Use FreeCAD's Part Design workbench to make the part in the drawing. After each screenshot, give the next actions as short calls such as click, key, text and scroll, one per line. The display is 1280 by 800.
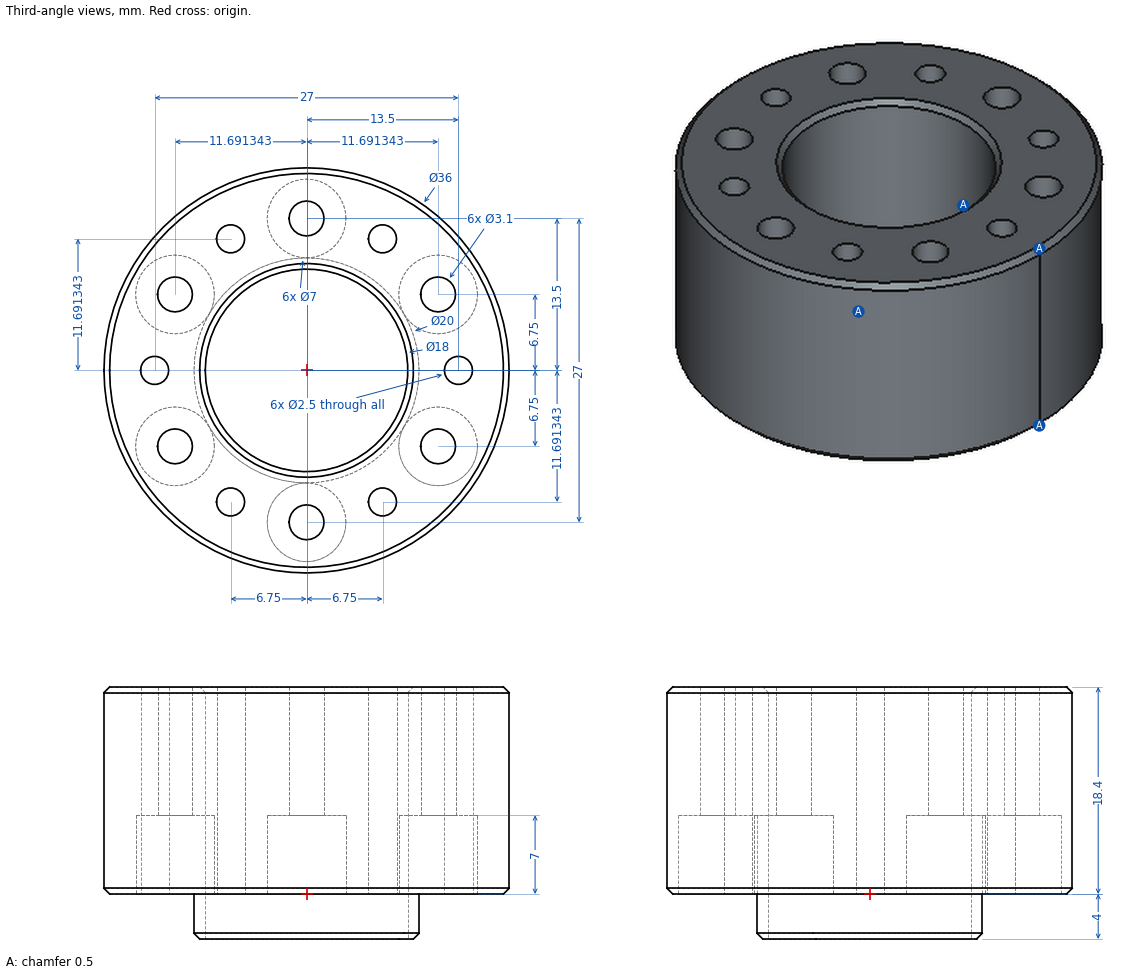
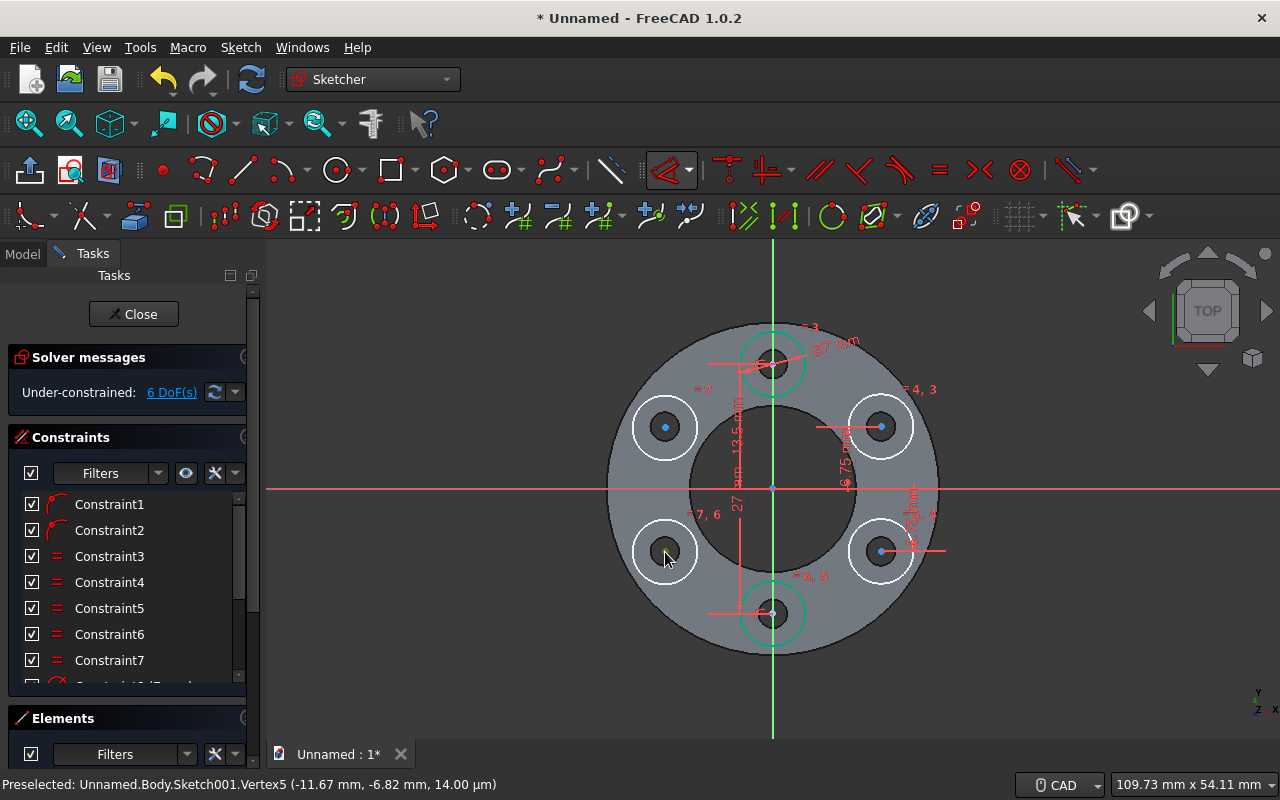
click(692, 170)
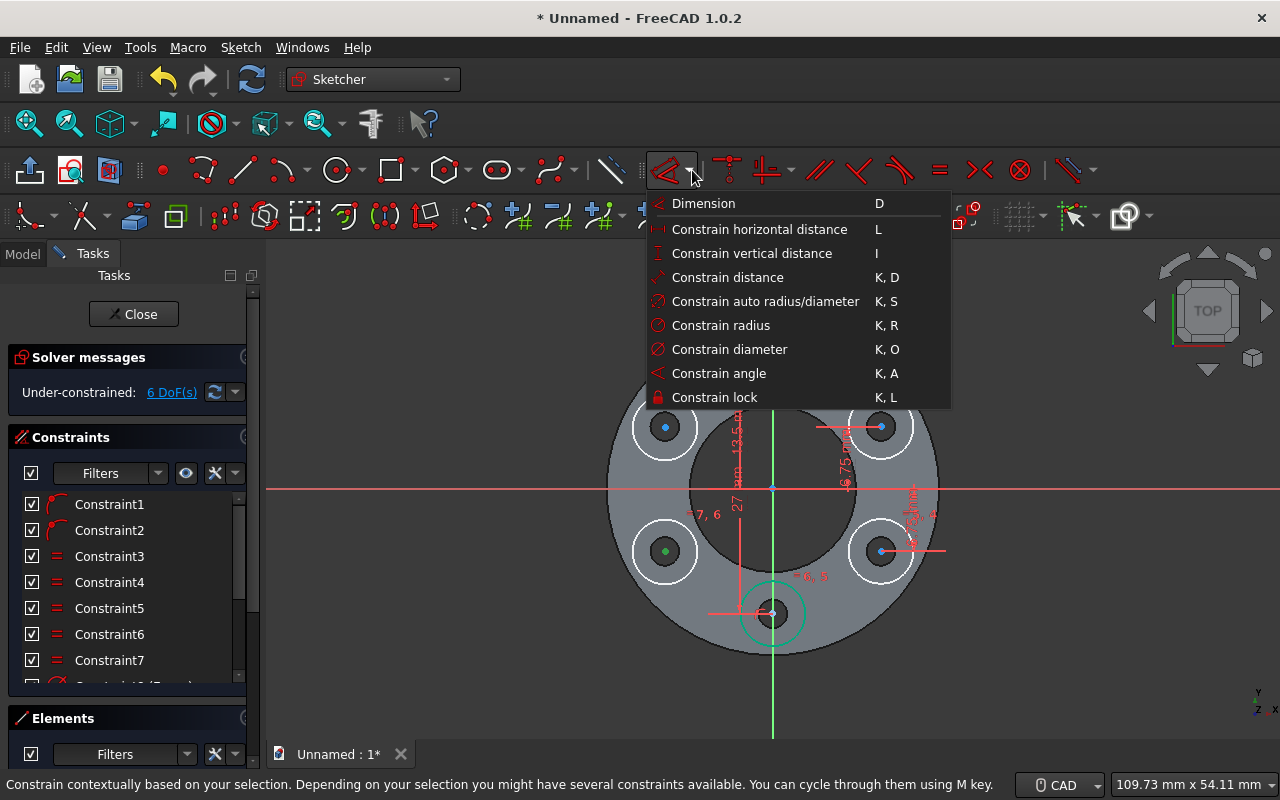
click(799, 253)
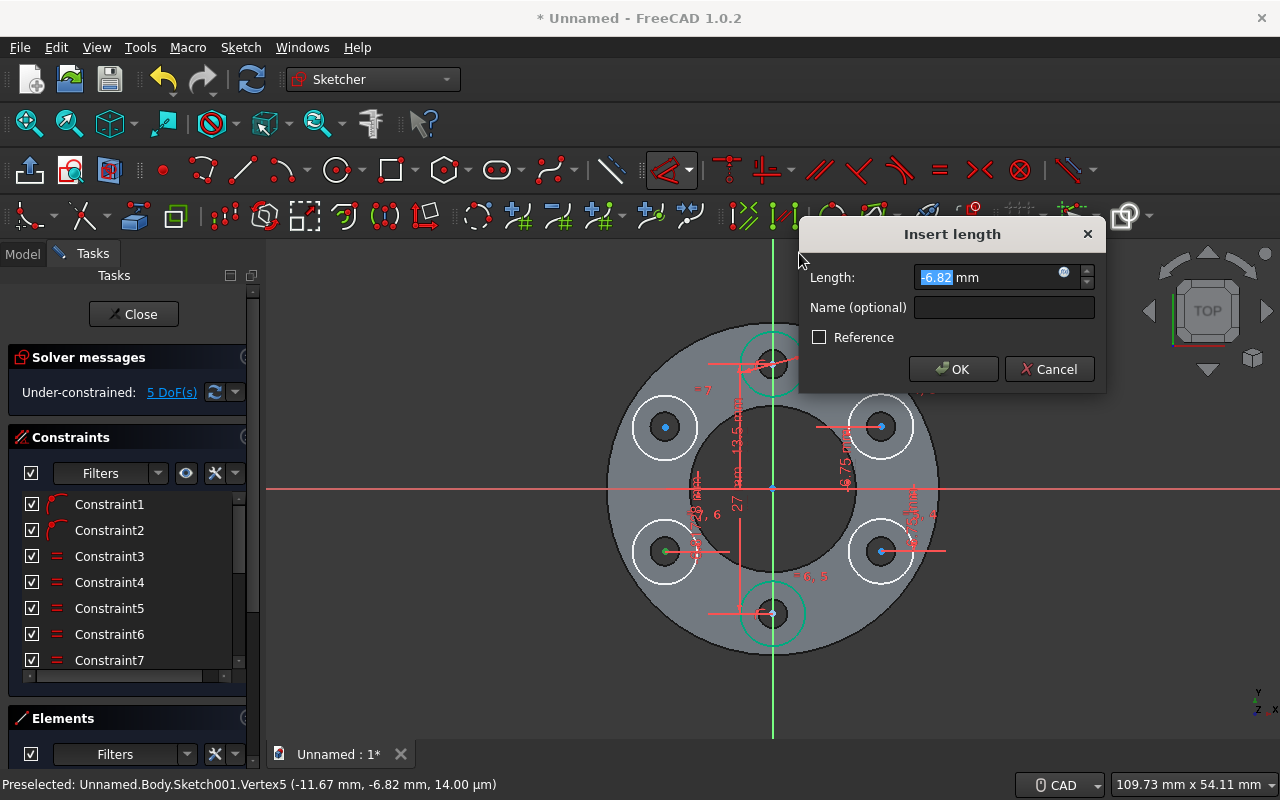
text(-6.75)
key(Return)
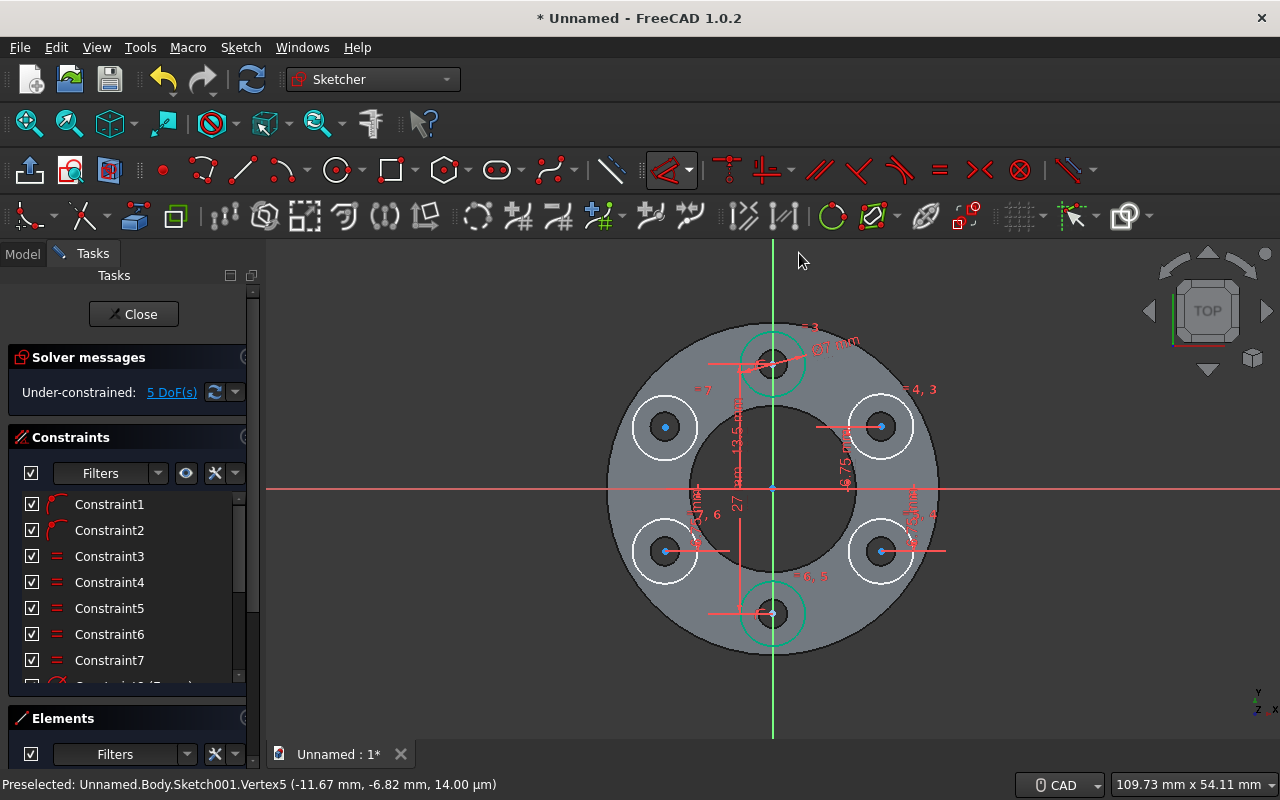
click(665, 428)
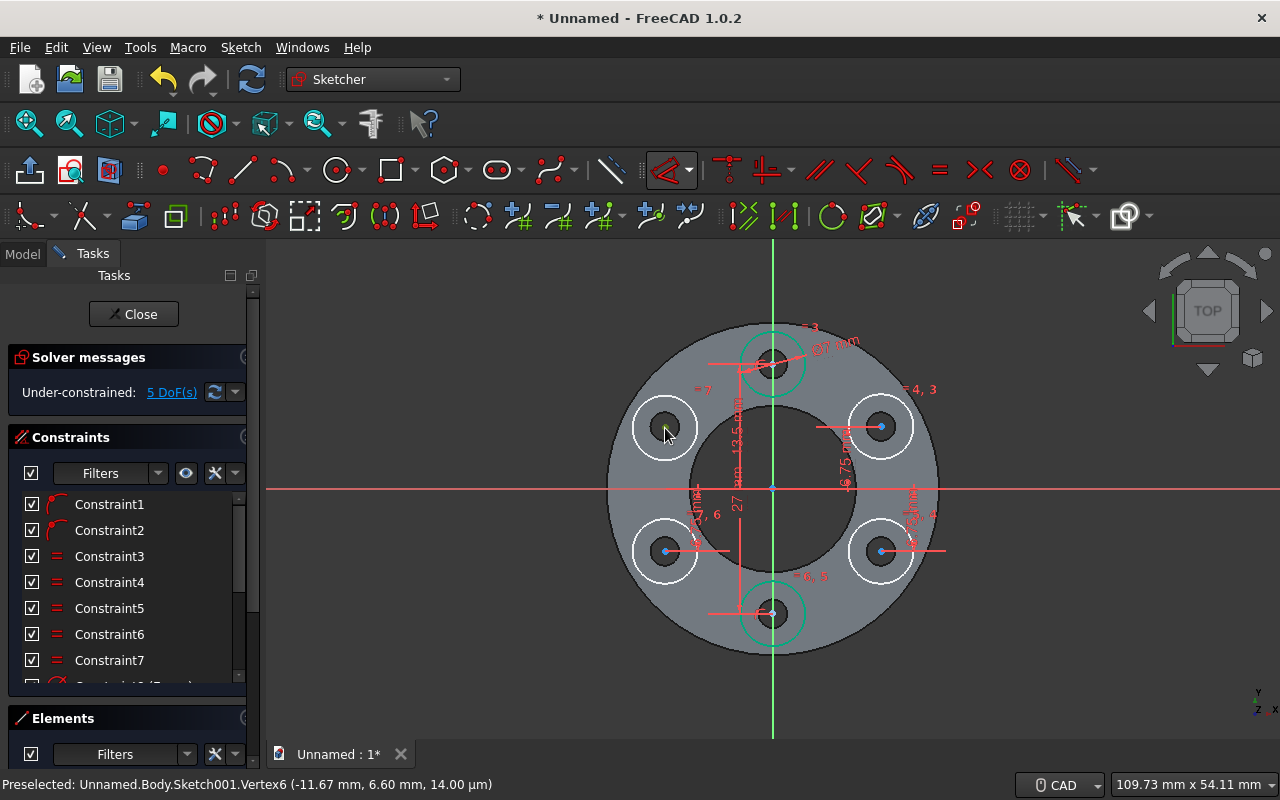
key(i)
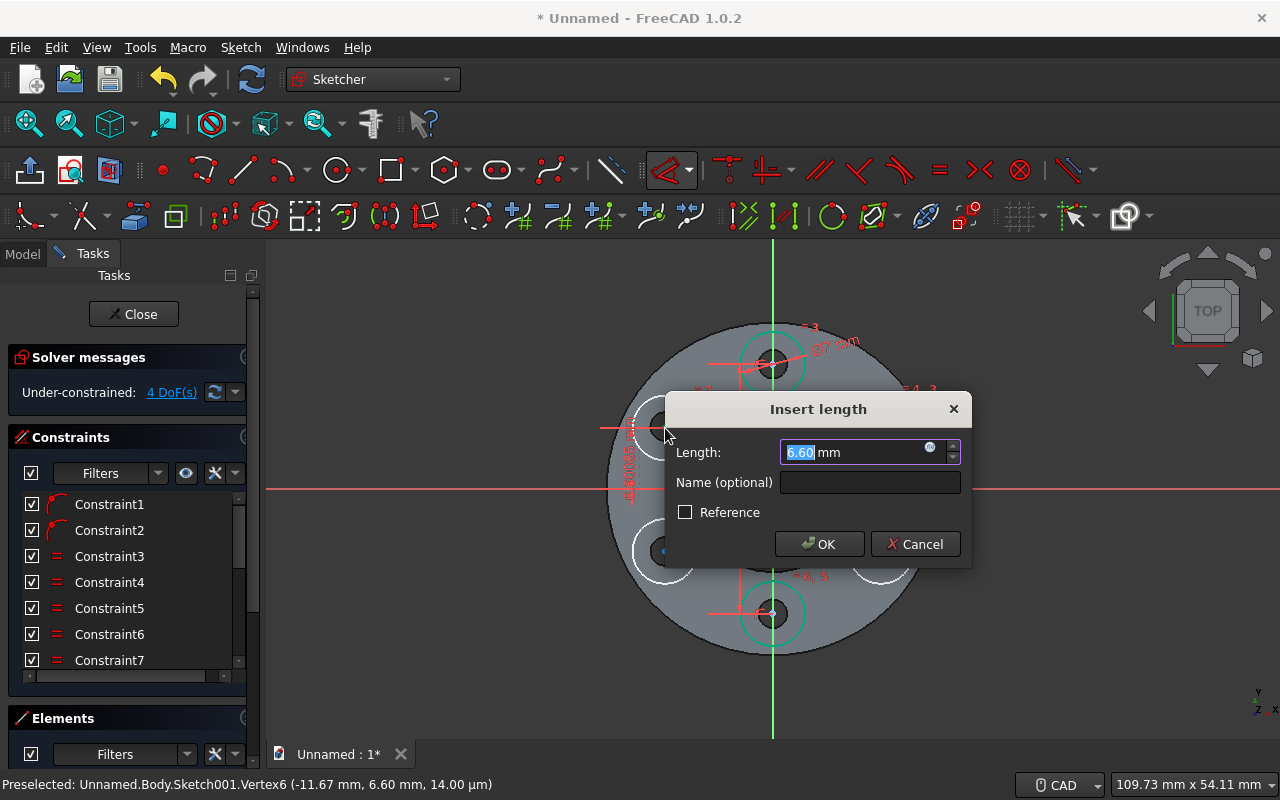
text(6.75)
key(Return)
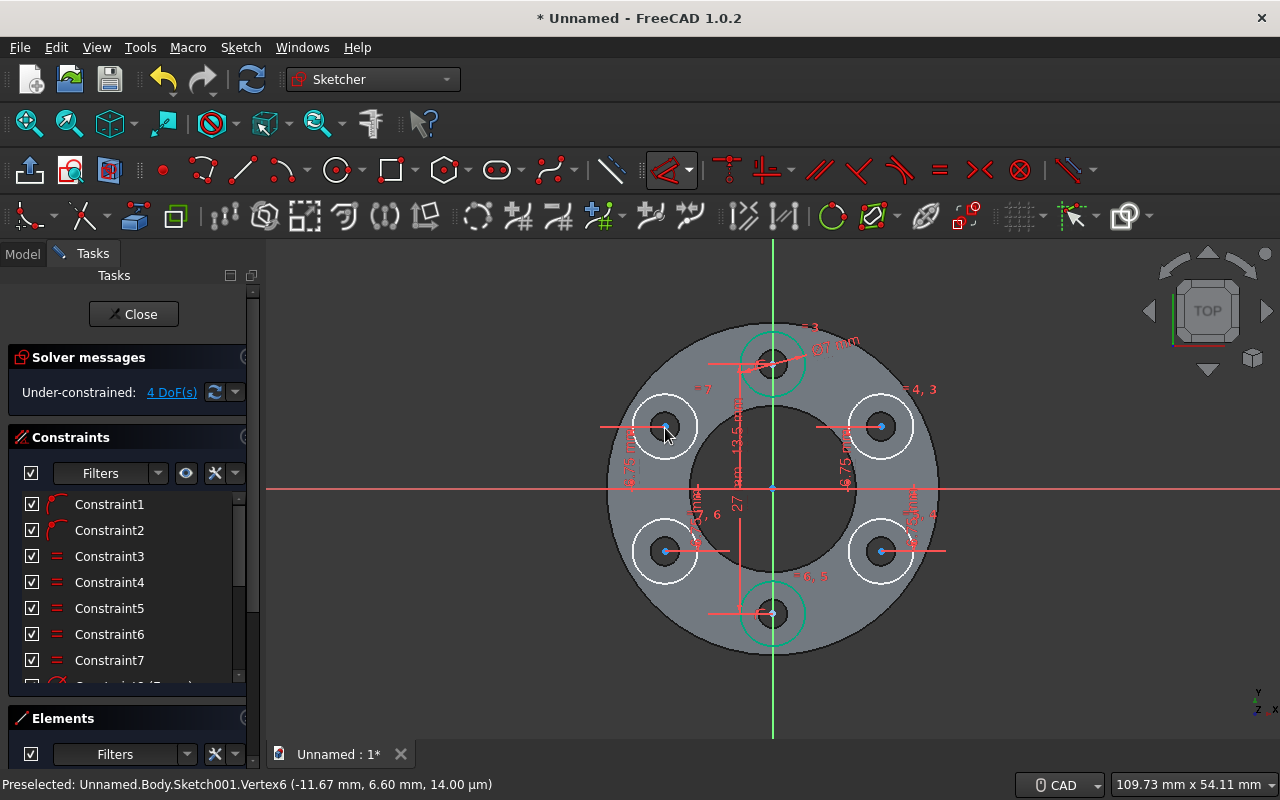
click(881, 427)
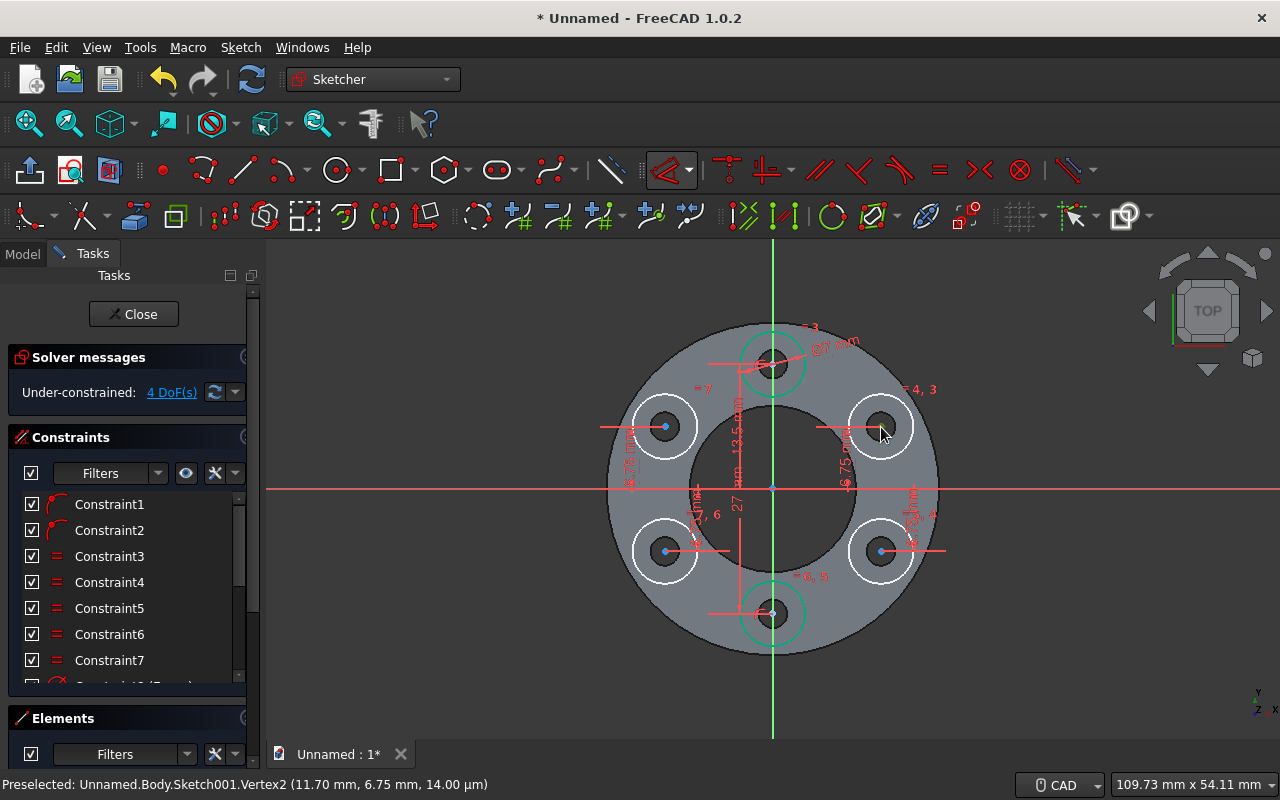
click(692, 170)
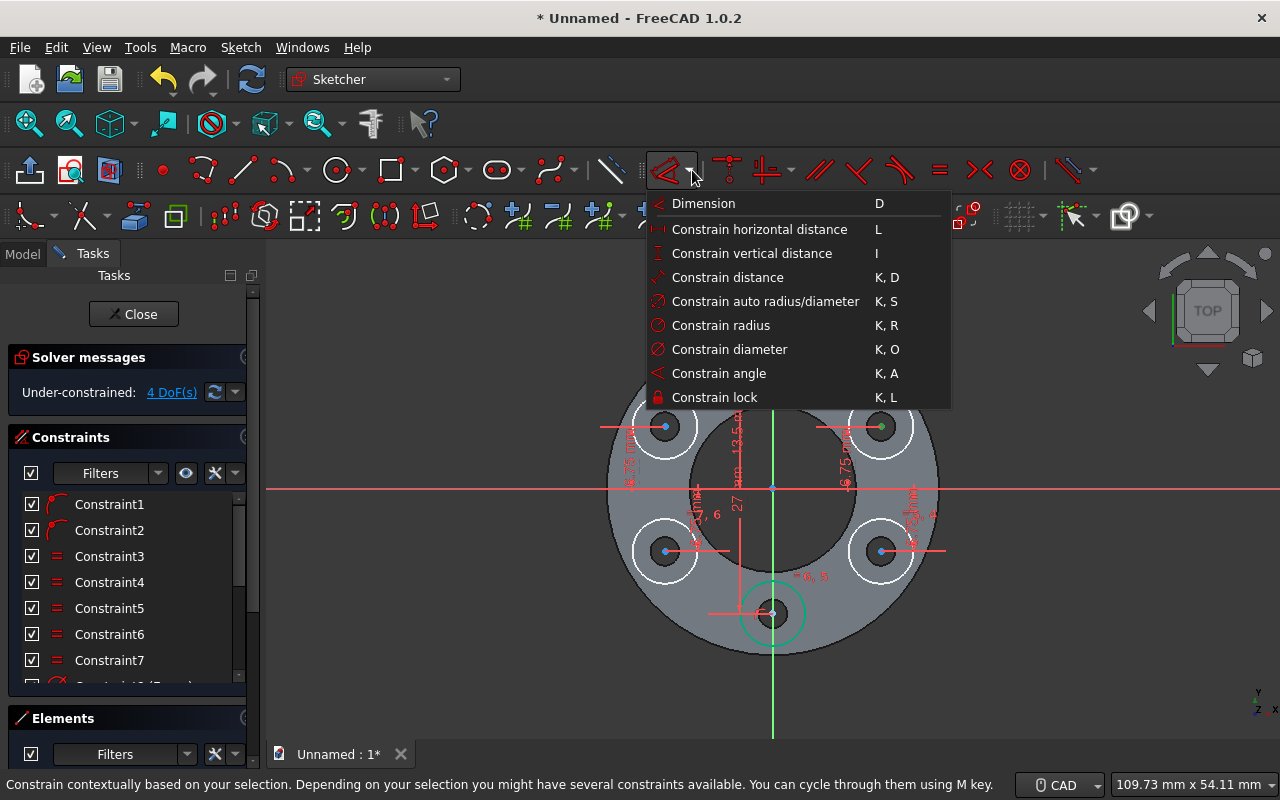
click(799, 229)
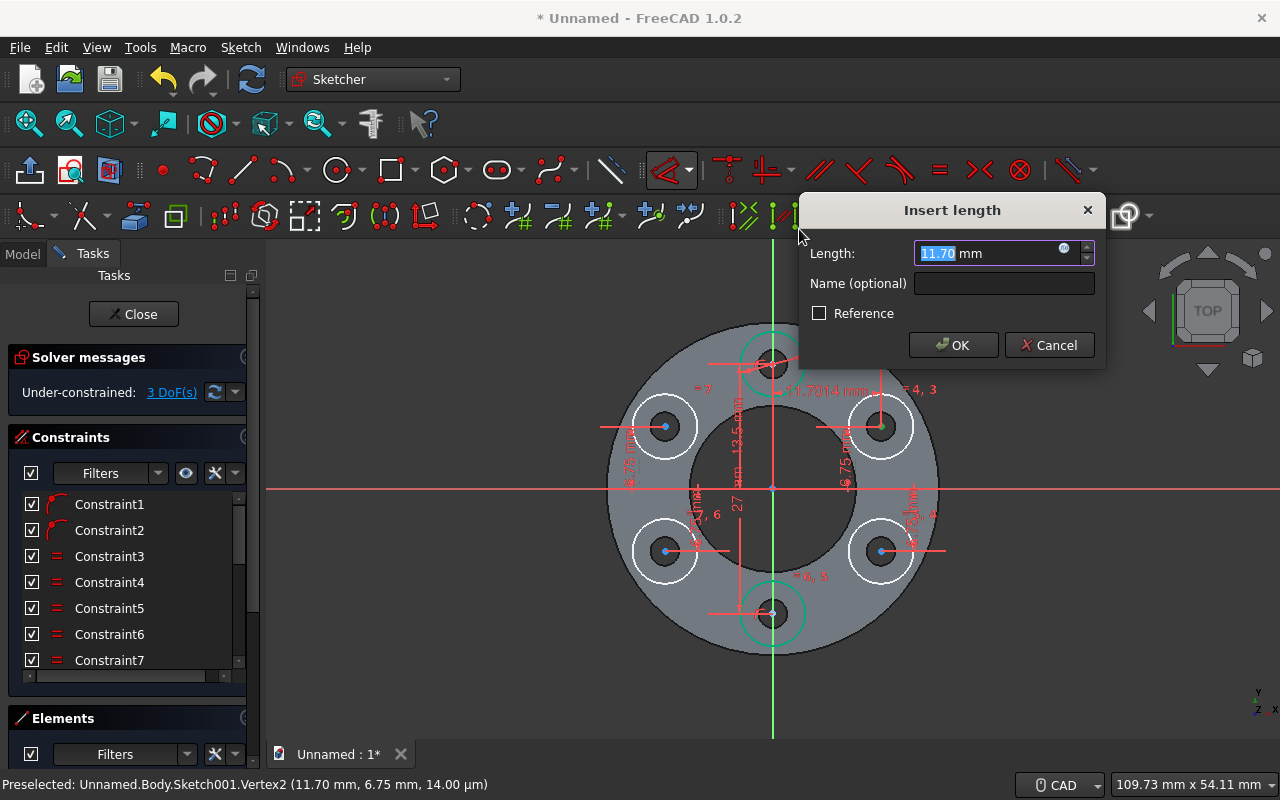
text(11.691343)
key(Return)